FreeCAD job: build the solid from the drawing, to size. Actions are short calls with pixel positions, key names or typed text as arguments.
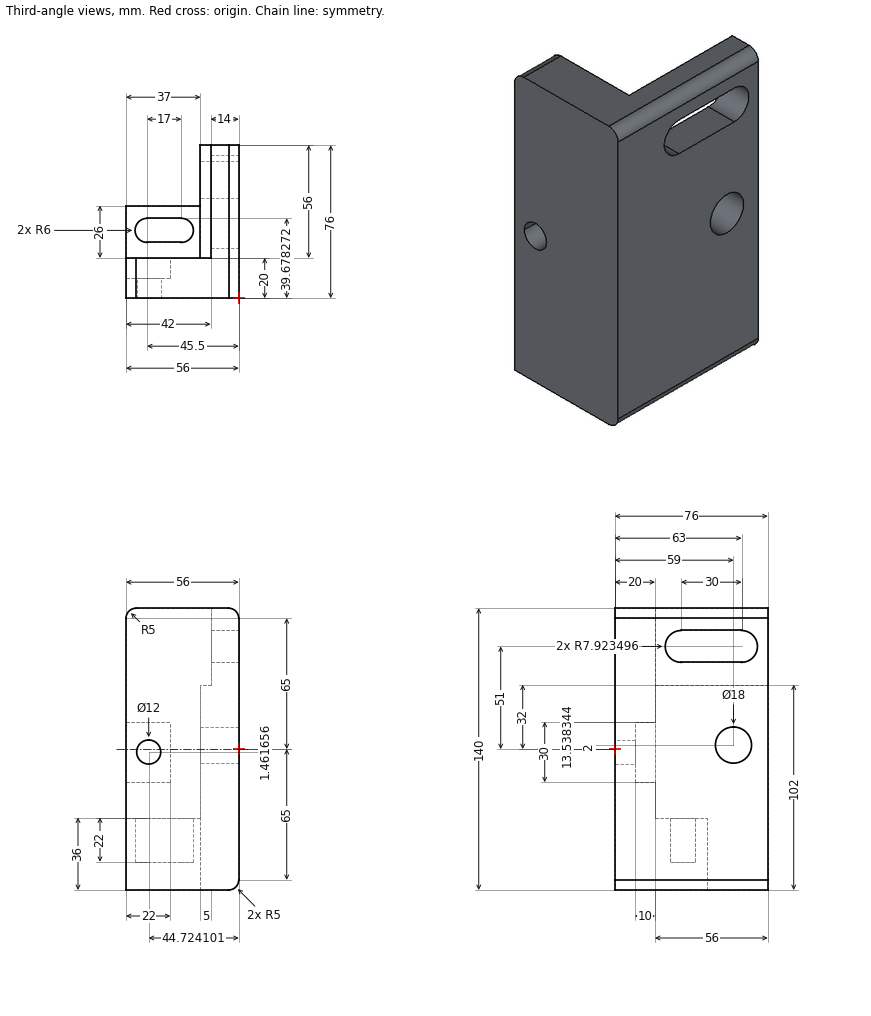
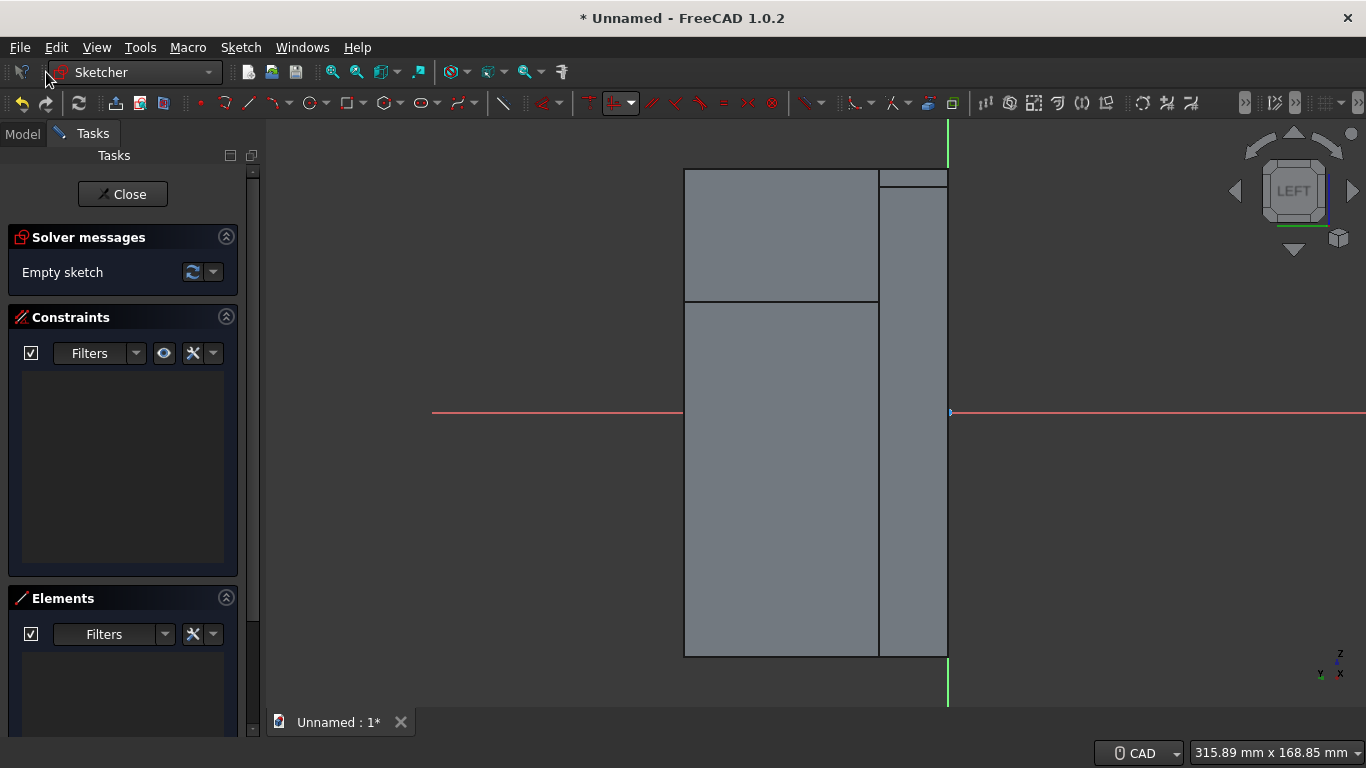
scroll(919, 186, up, 3)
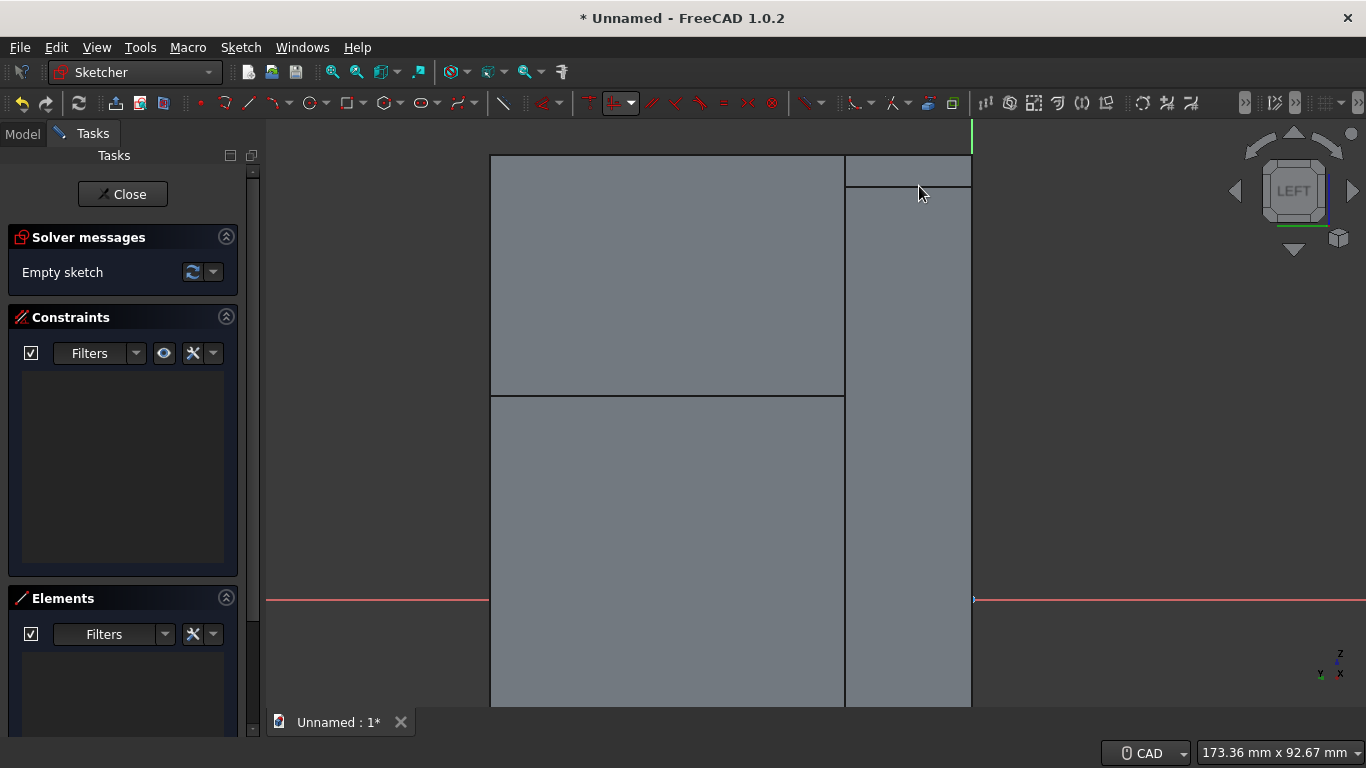
click(422, 104)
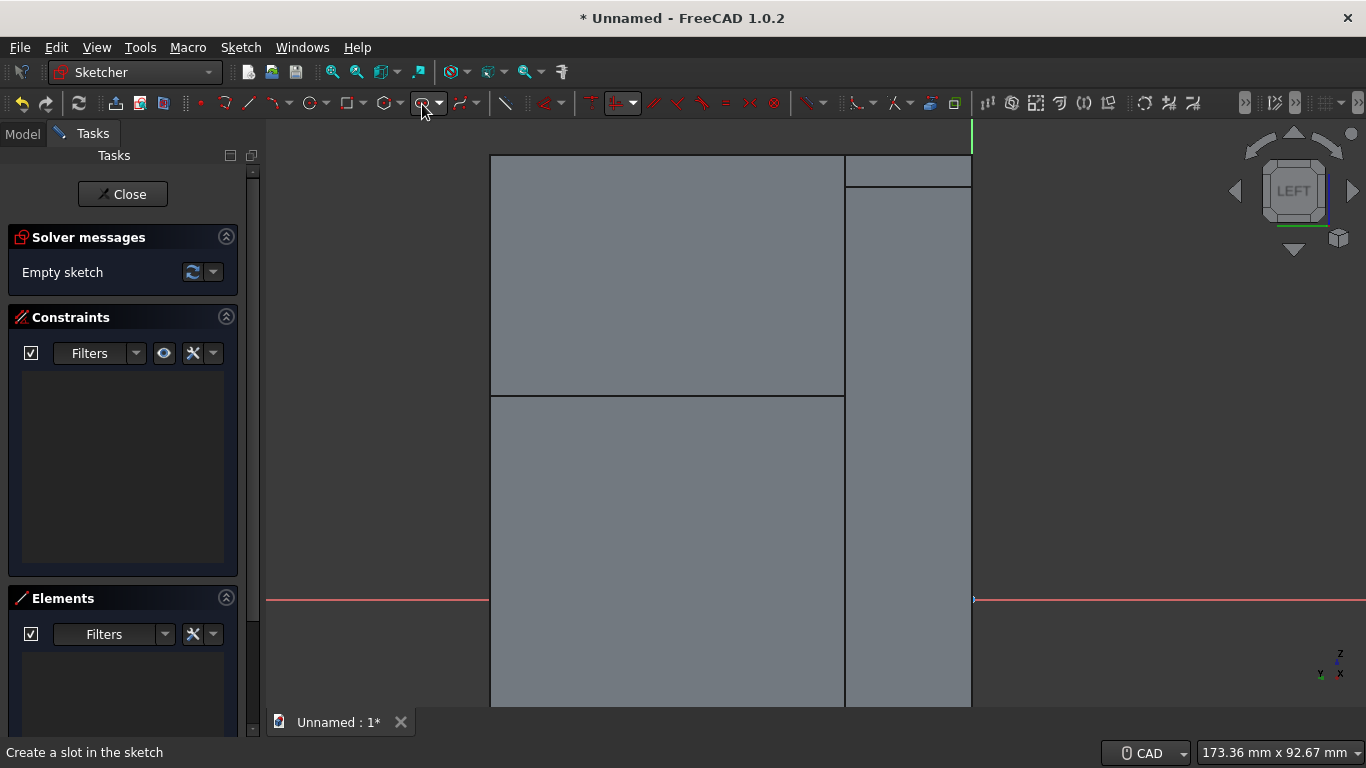
click(572, 276)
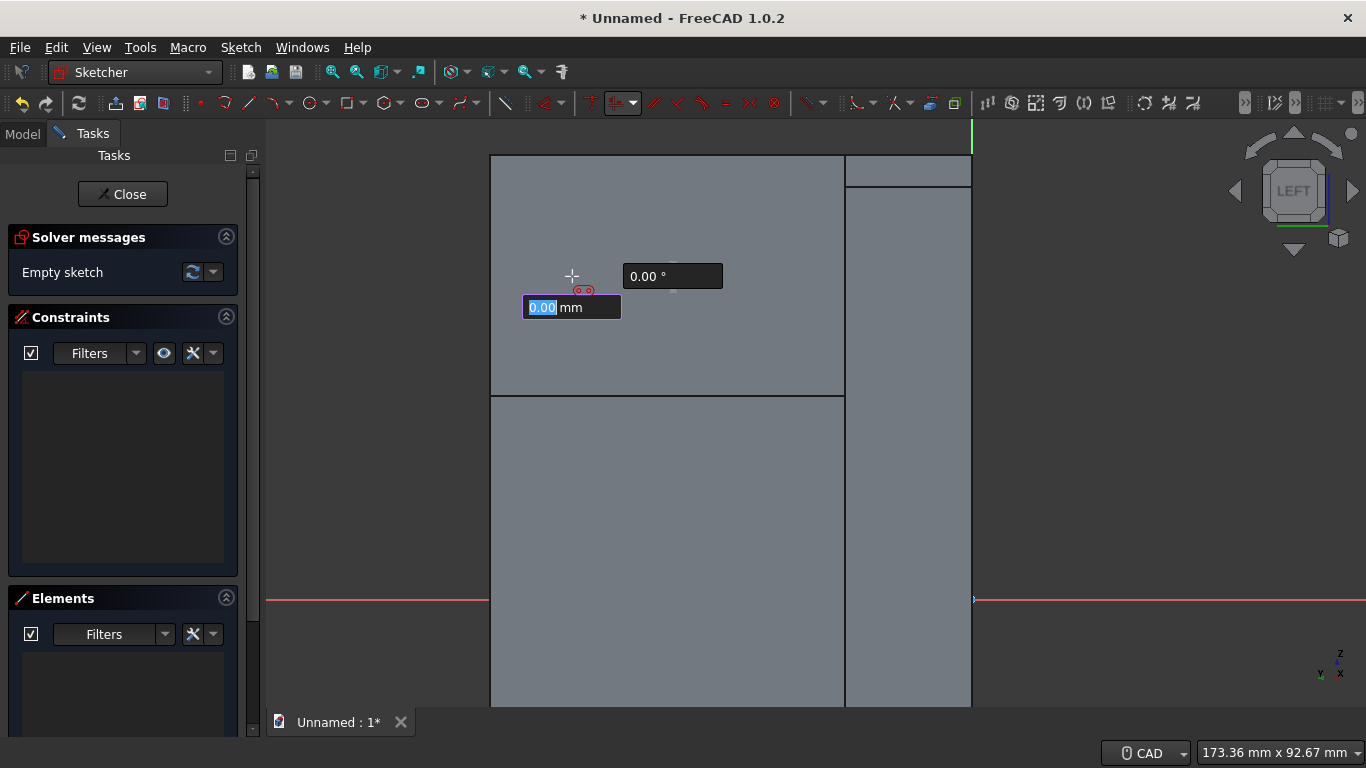
click(763, 276)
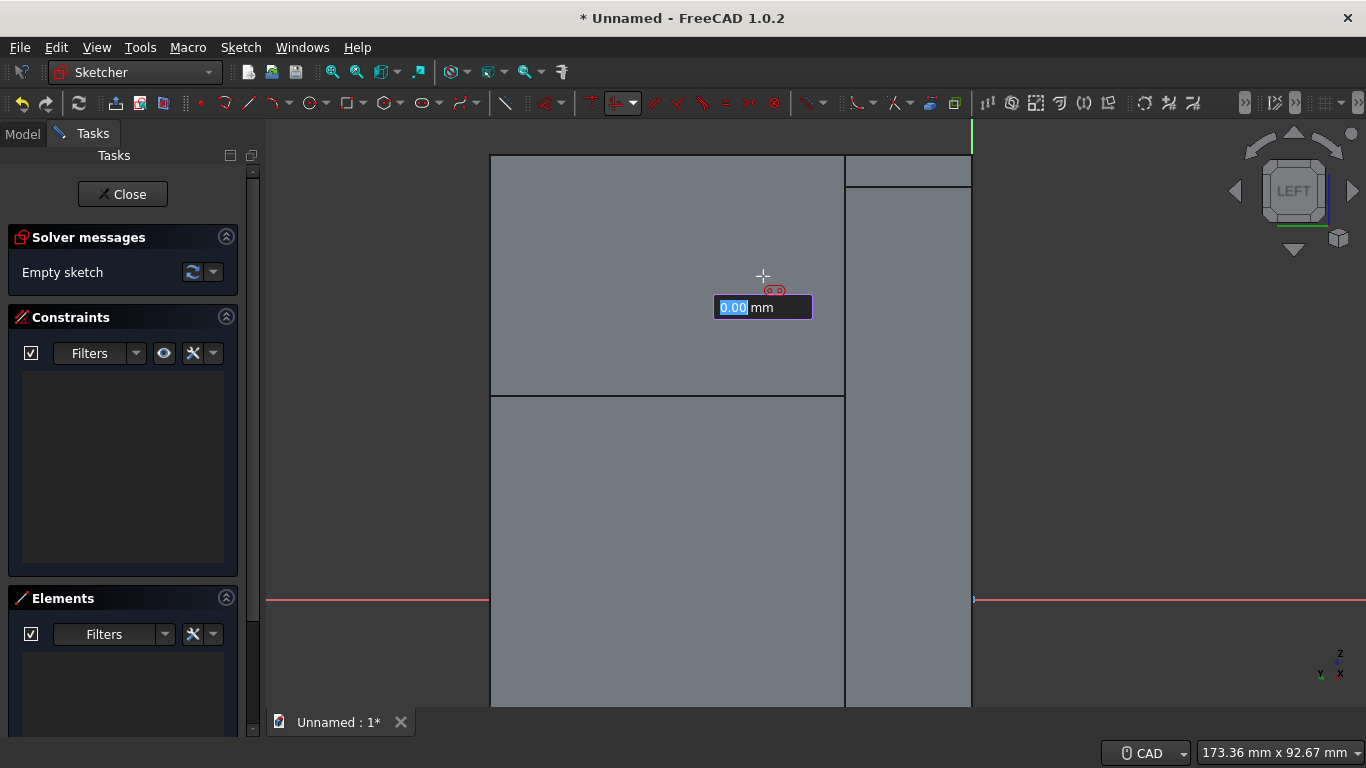
click(667, 326)
key(Escape)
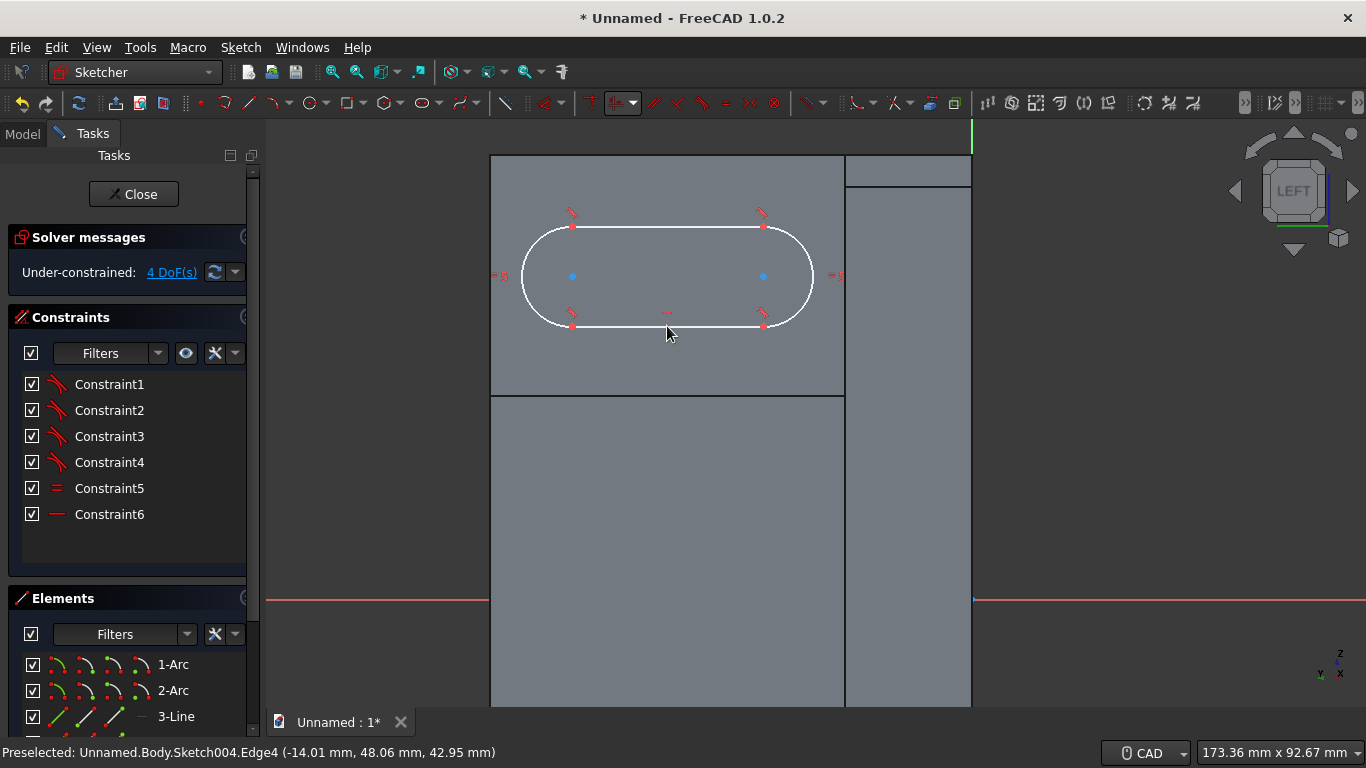
key(d)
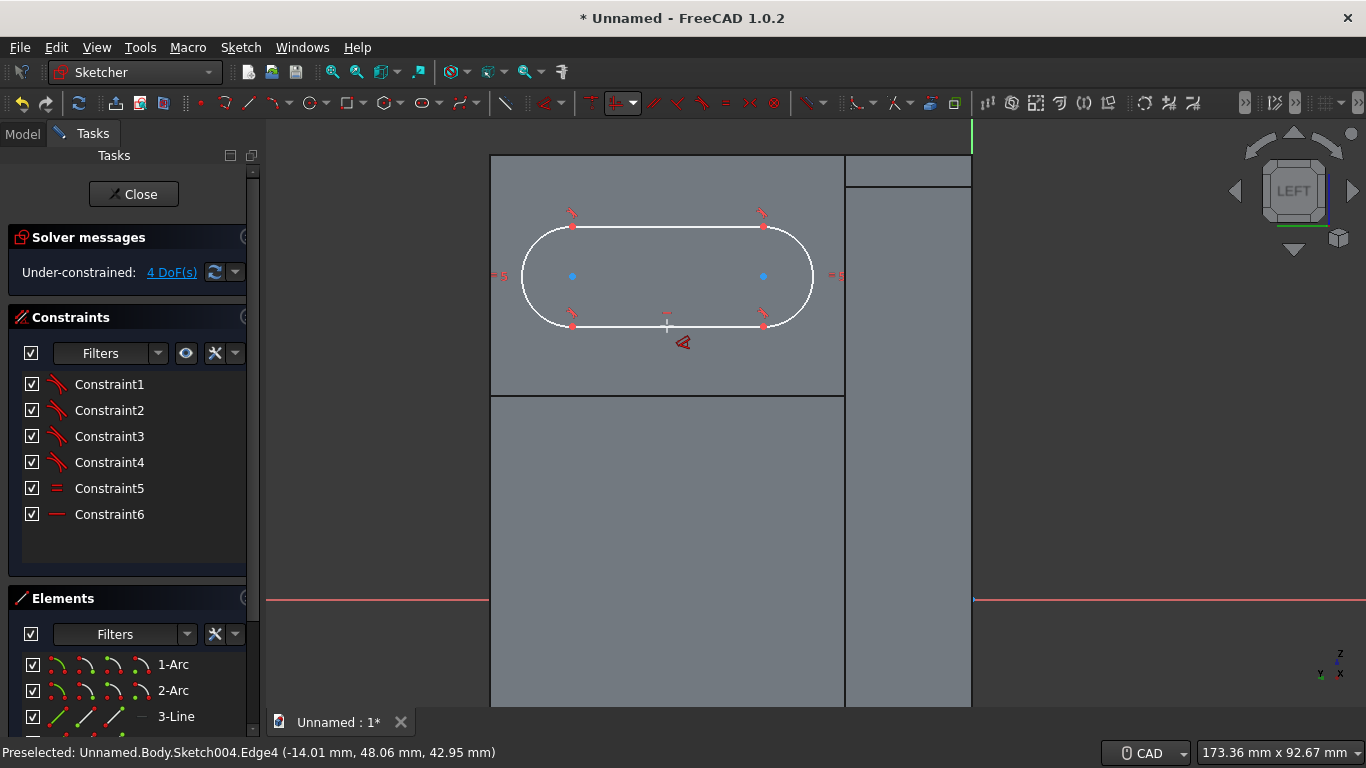
click(532, 248)
click(506, 229)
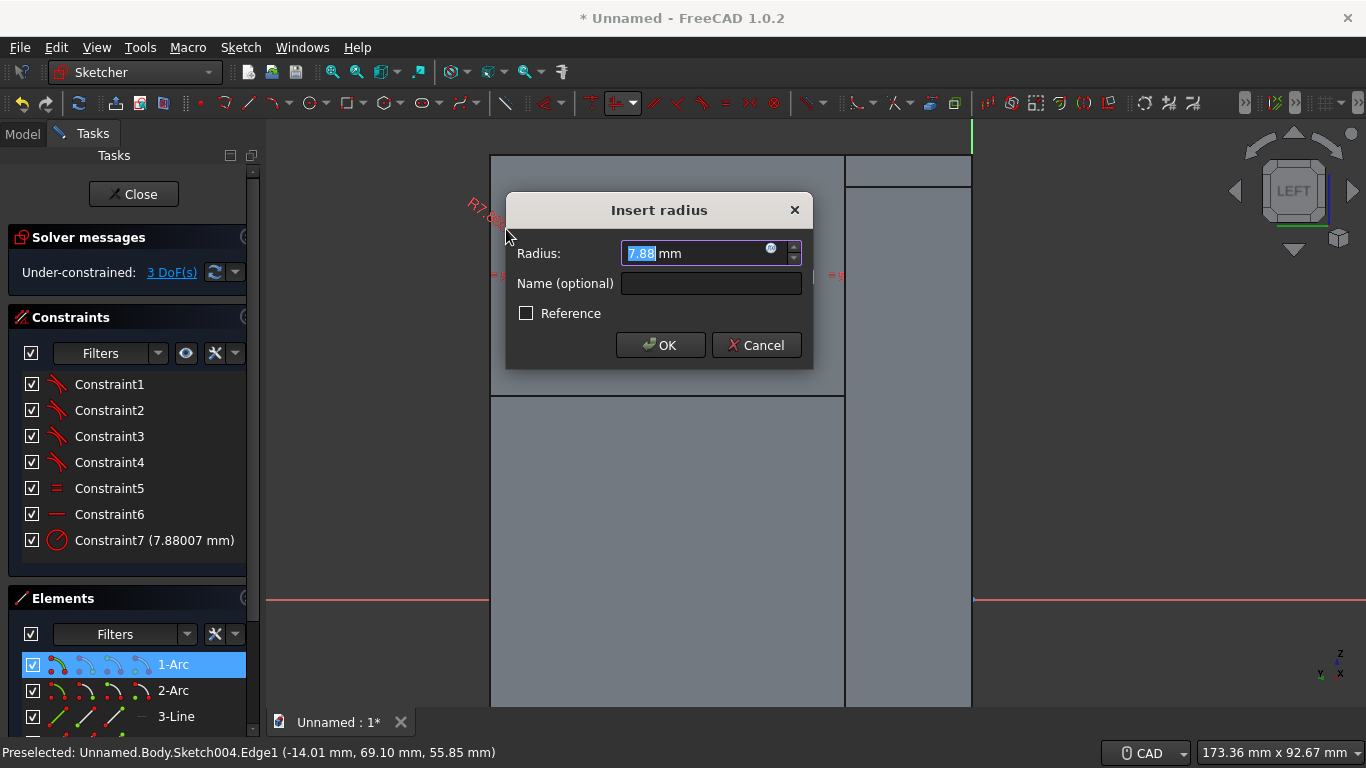
text(7.923496)
key(Return)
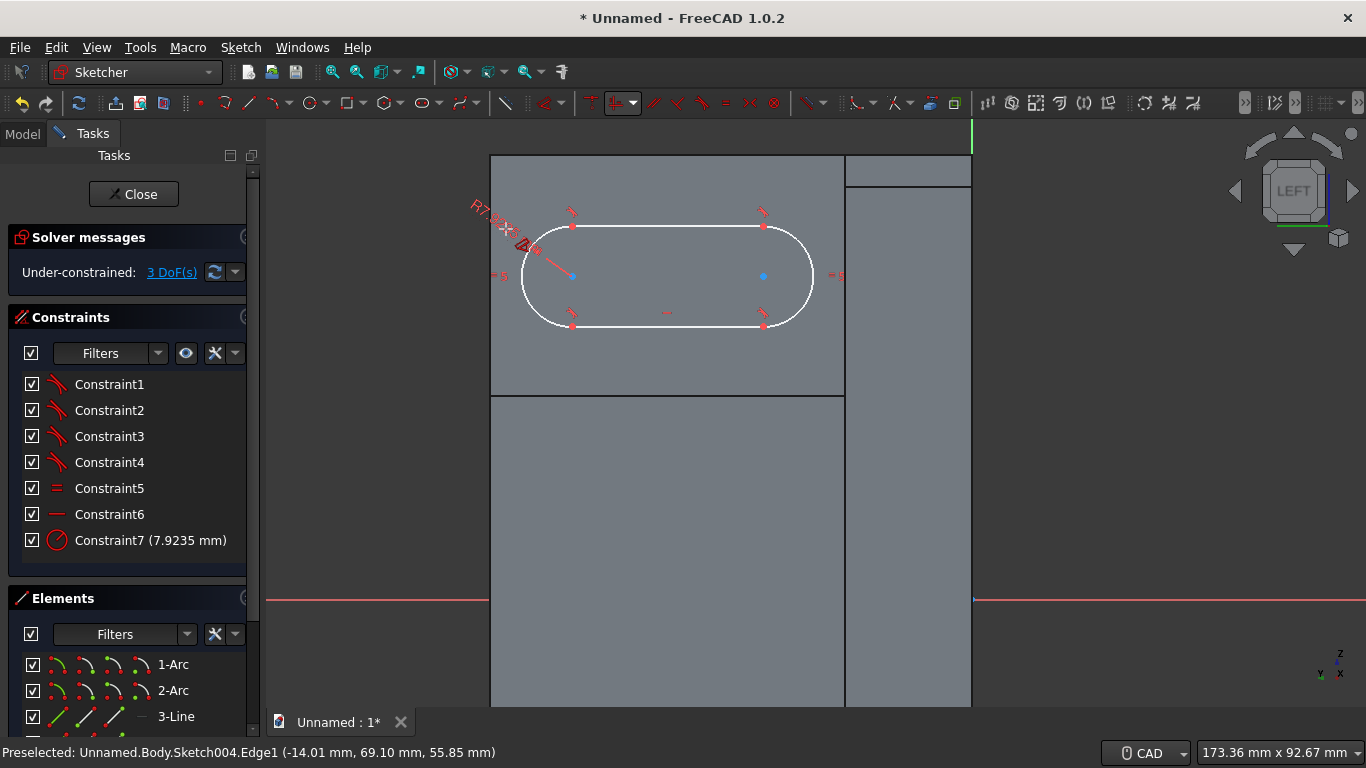
click(629, 226)
click(667, 192)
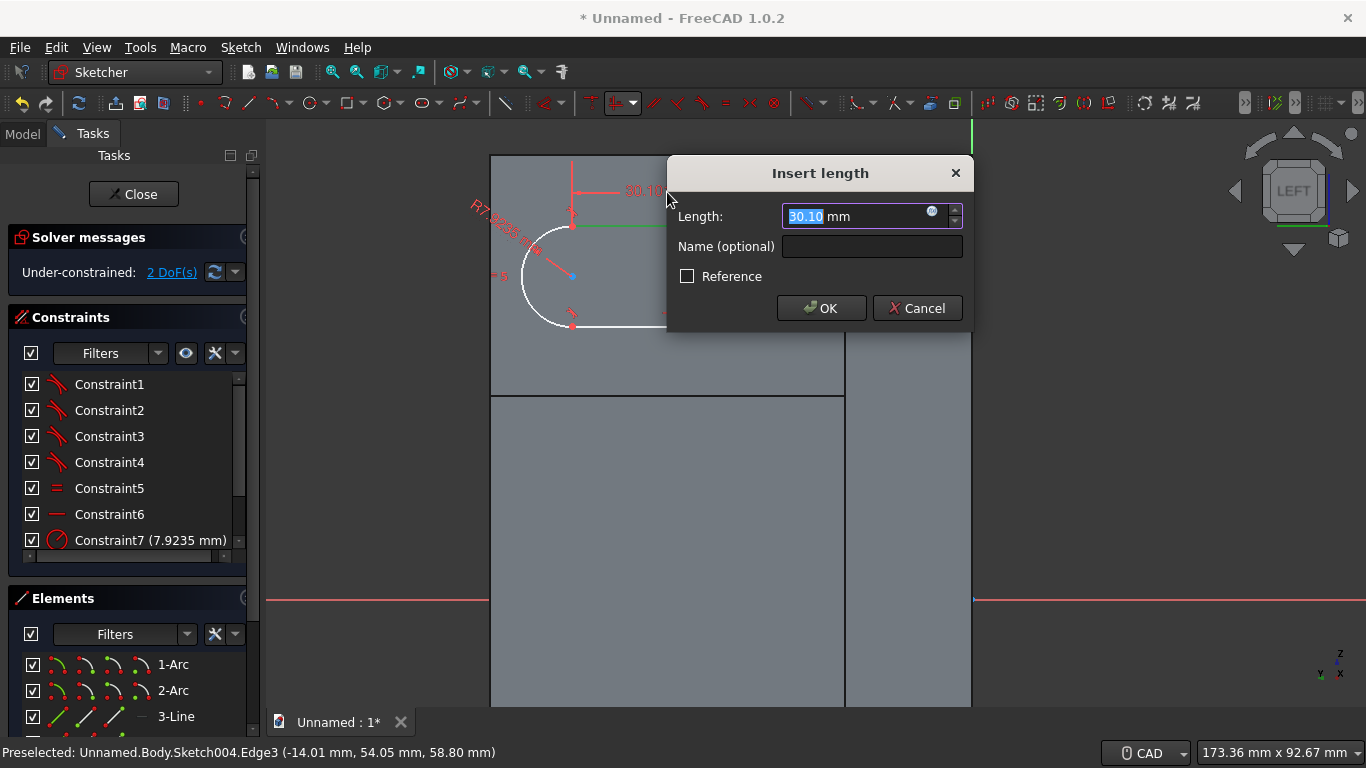
text(30)
key(Return)